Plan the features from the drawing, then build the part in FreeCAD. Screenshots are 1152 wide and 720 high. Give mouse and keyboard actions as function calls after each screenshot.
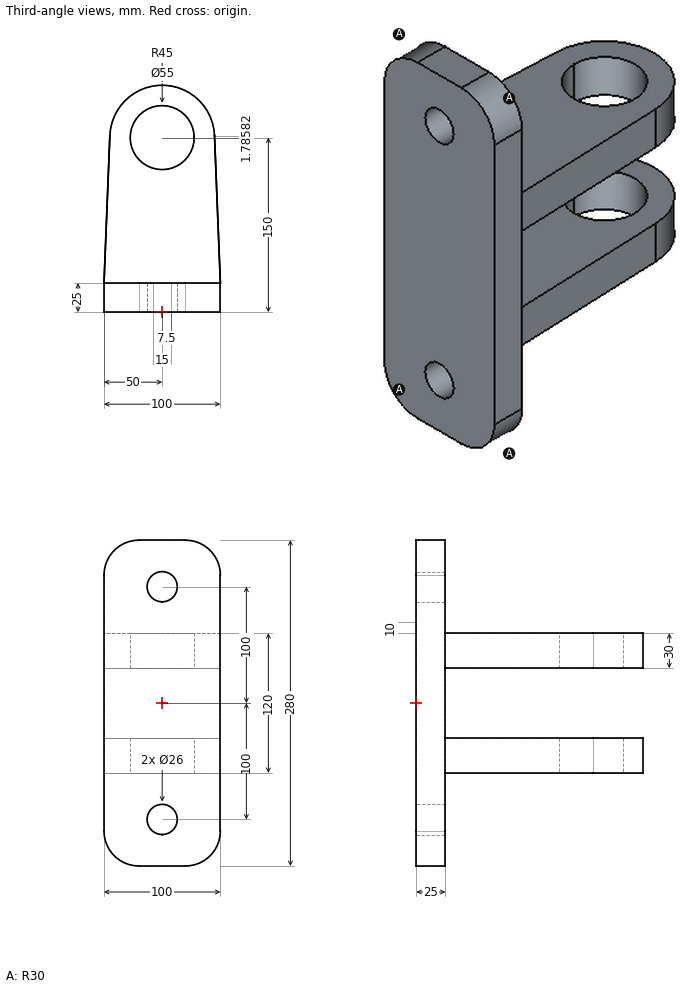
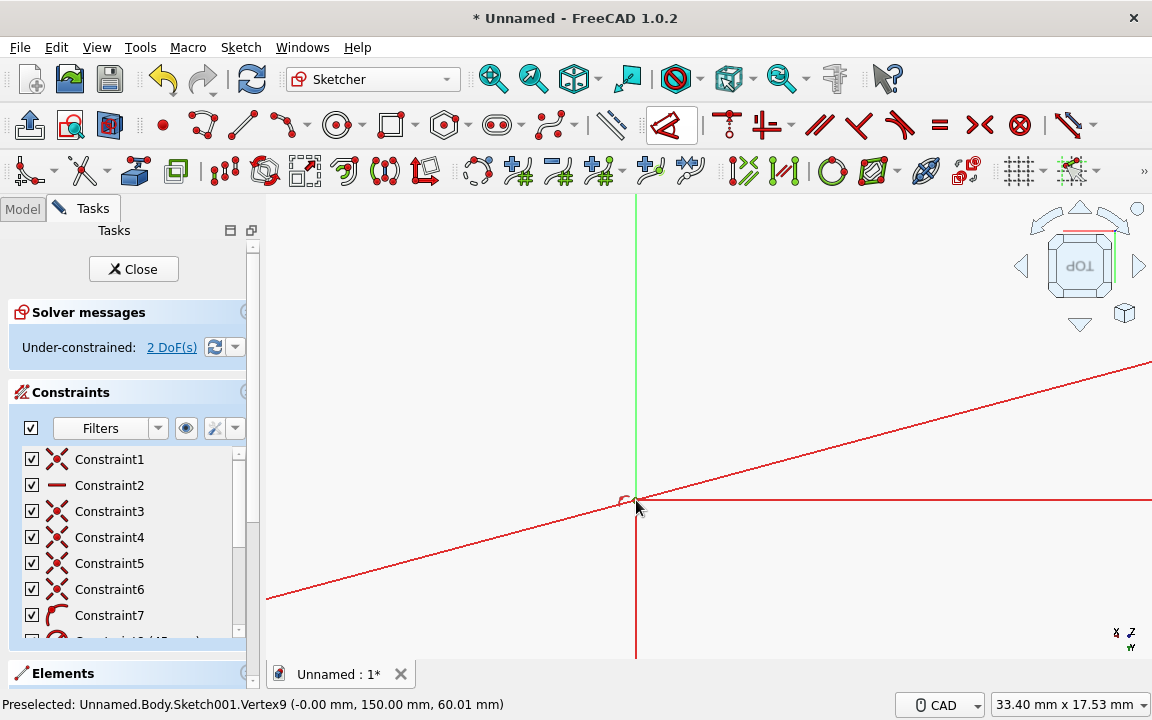
click(692, 126)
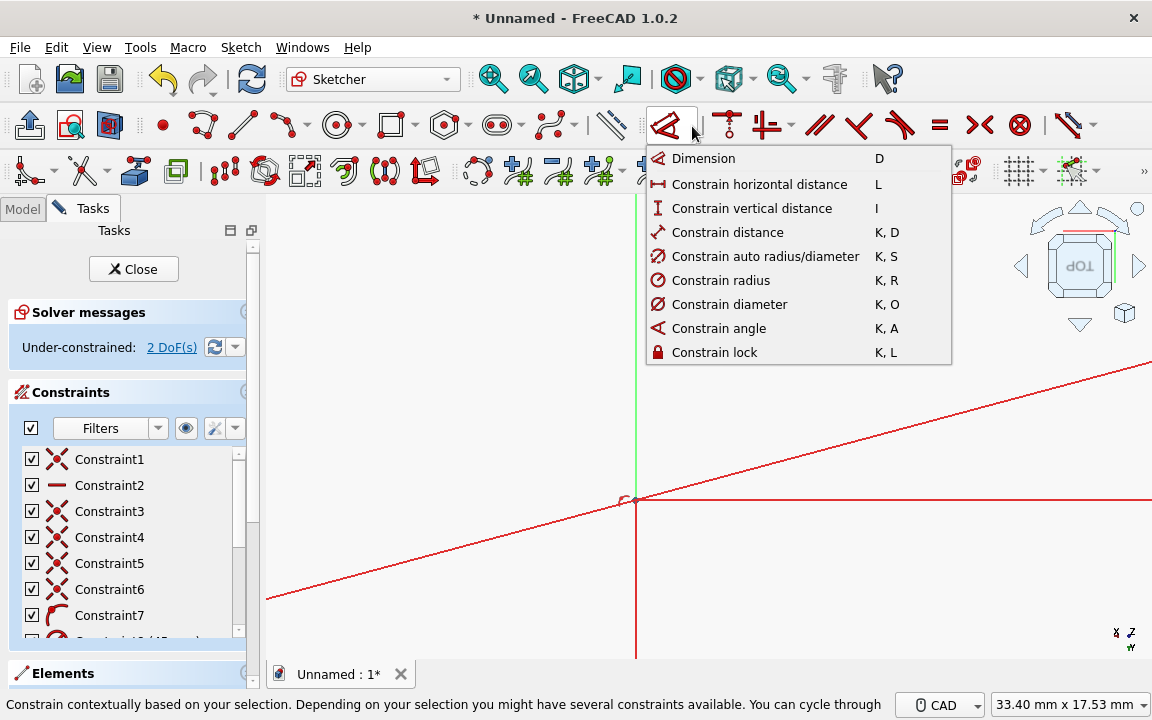
click(799, 208)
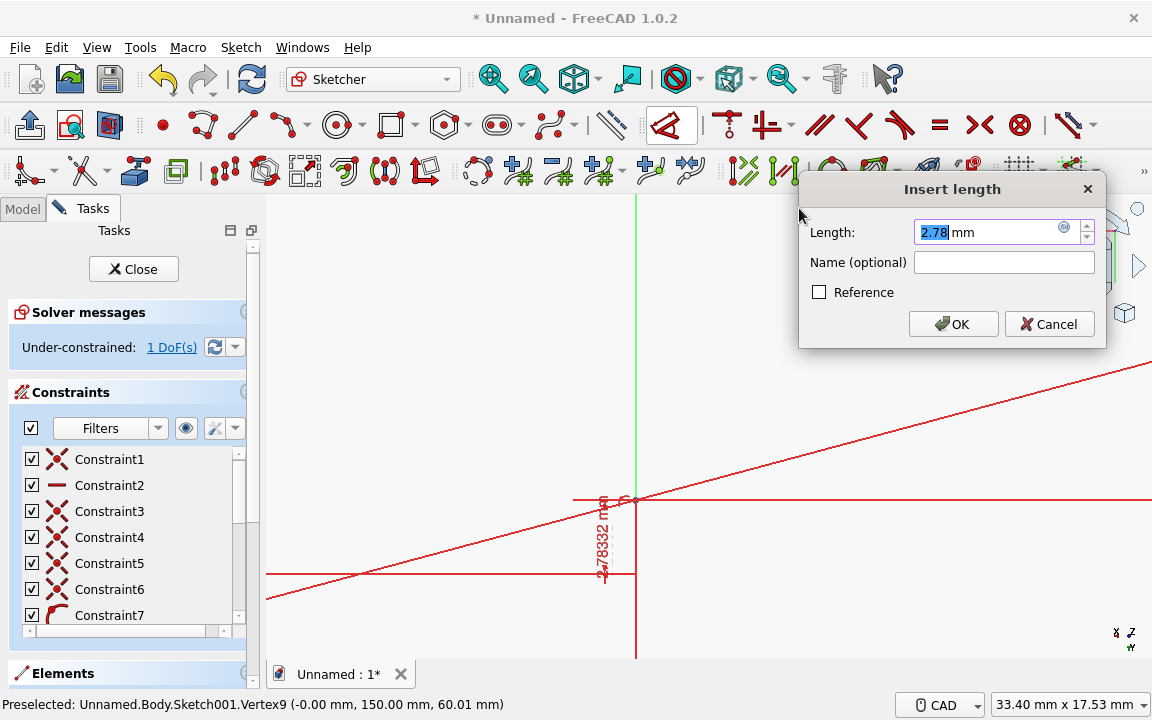
text(1.78582)
key(Return)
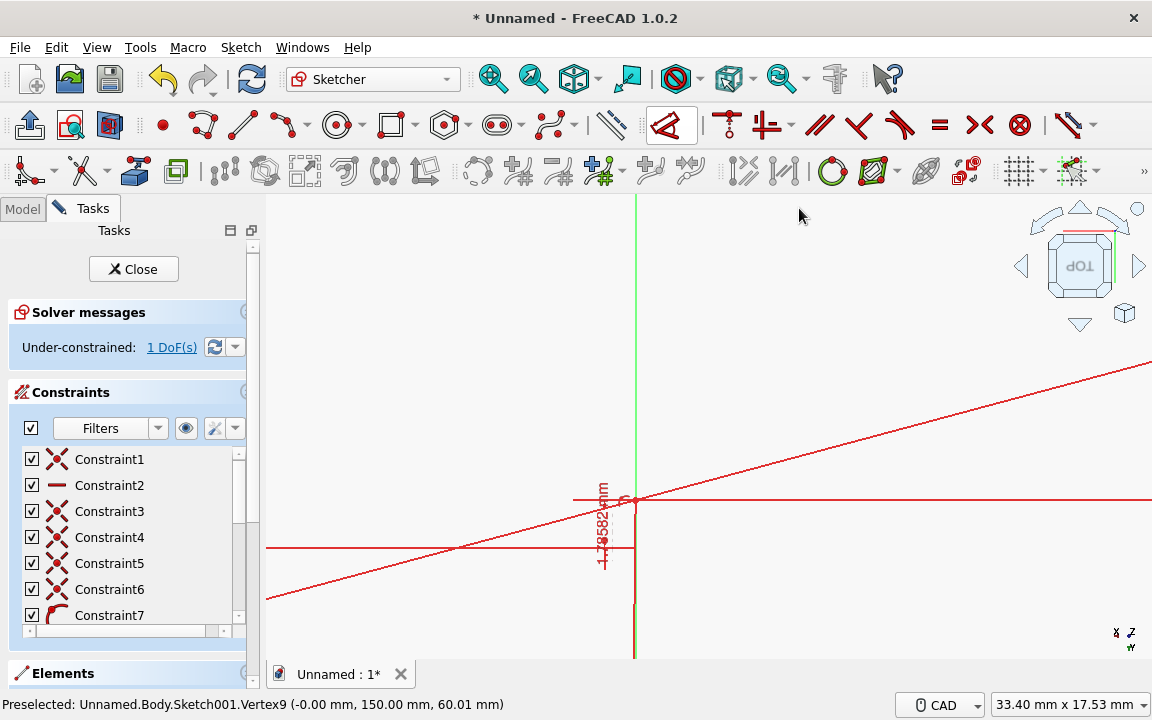
scroll(641, 512, down, 14)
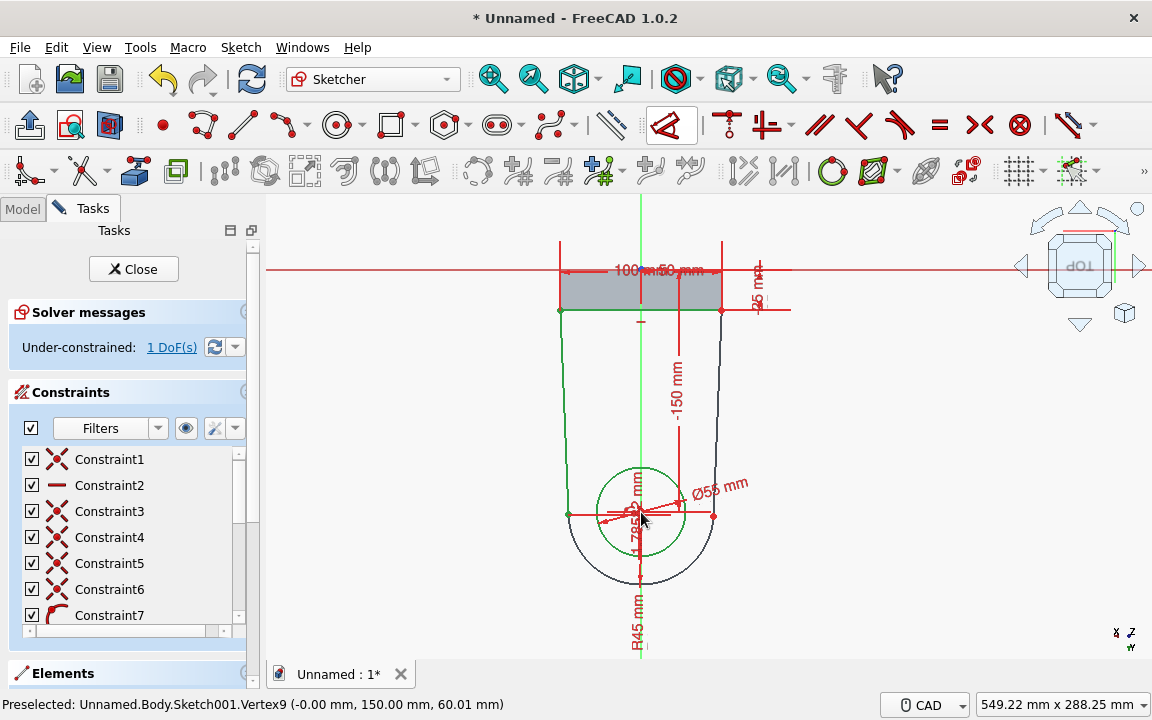
scroll(714, 516, up, 14)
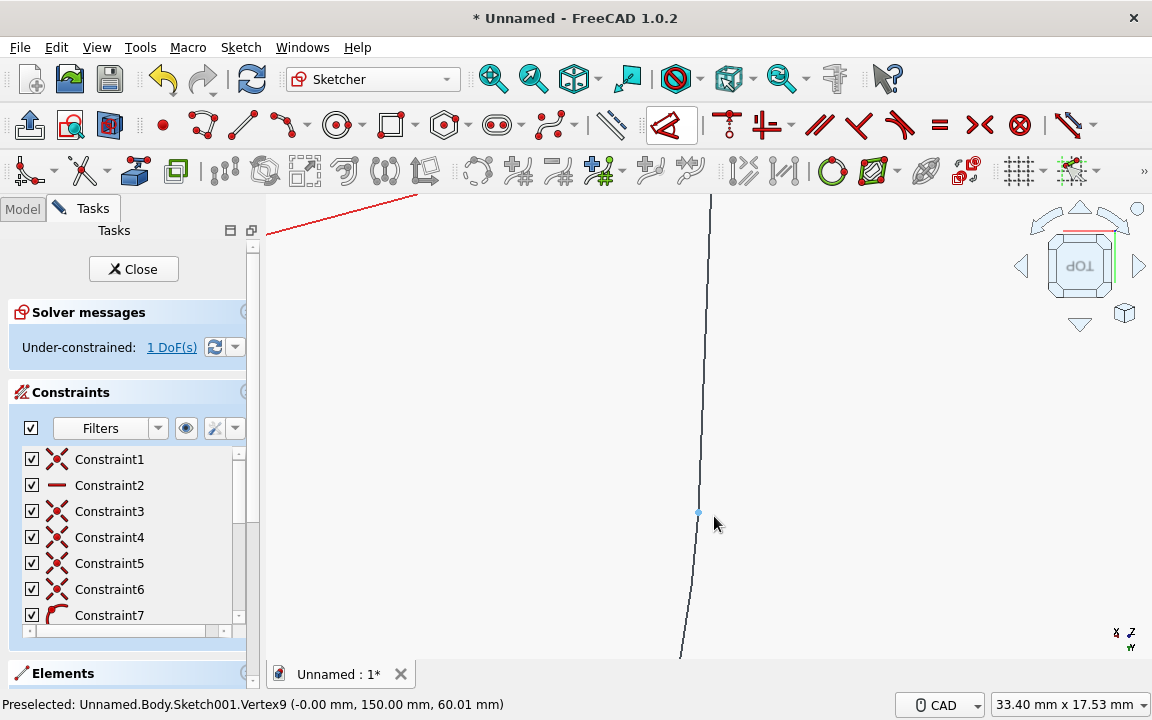
click(698, 512)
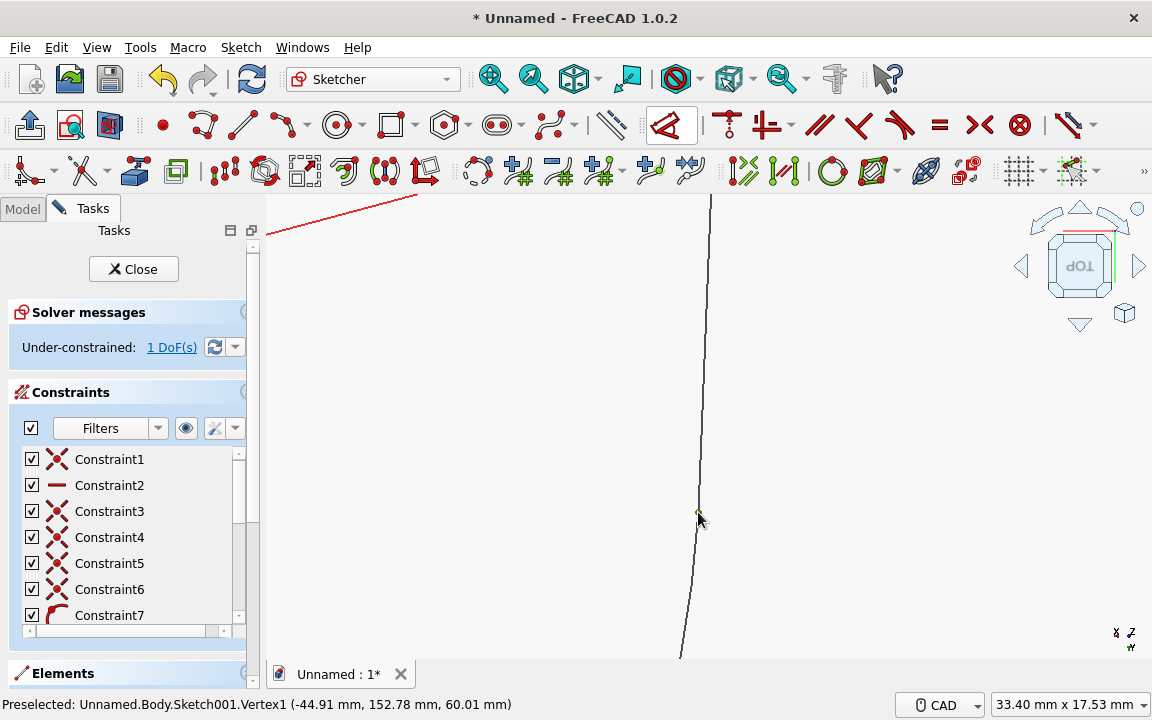
scroll(714, 516, down, 14)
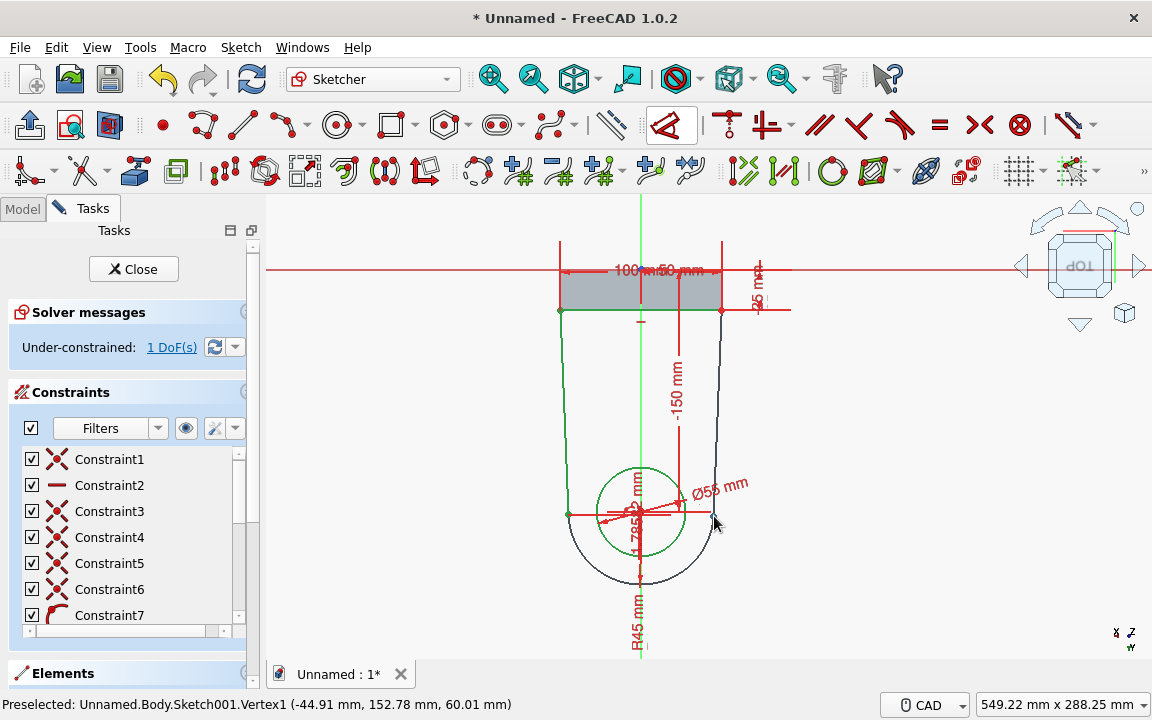
scroll(641, 512, up, 14)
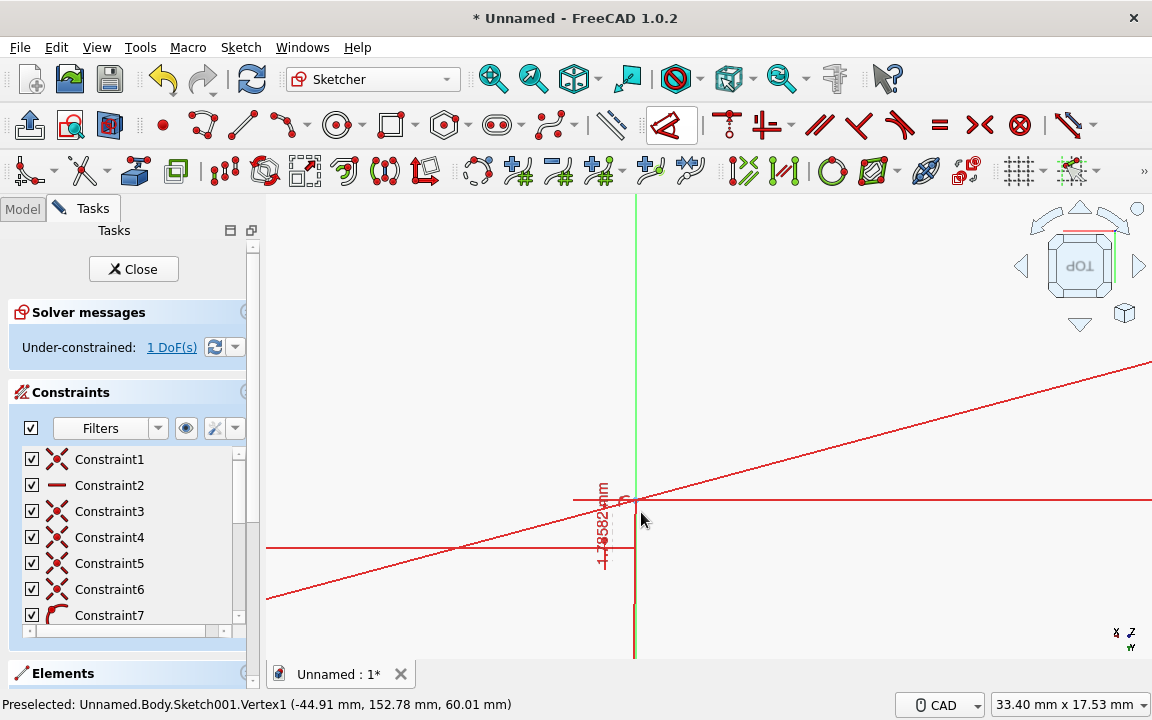
click(636, 500)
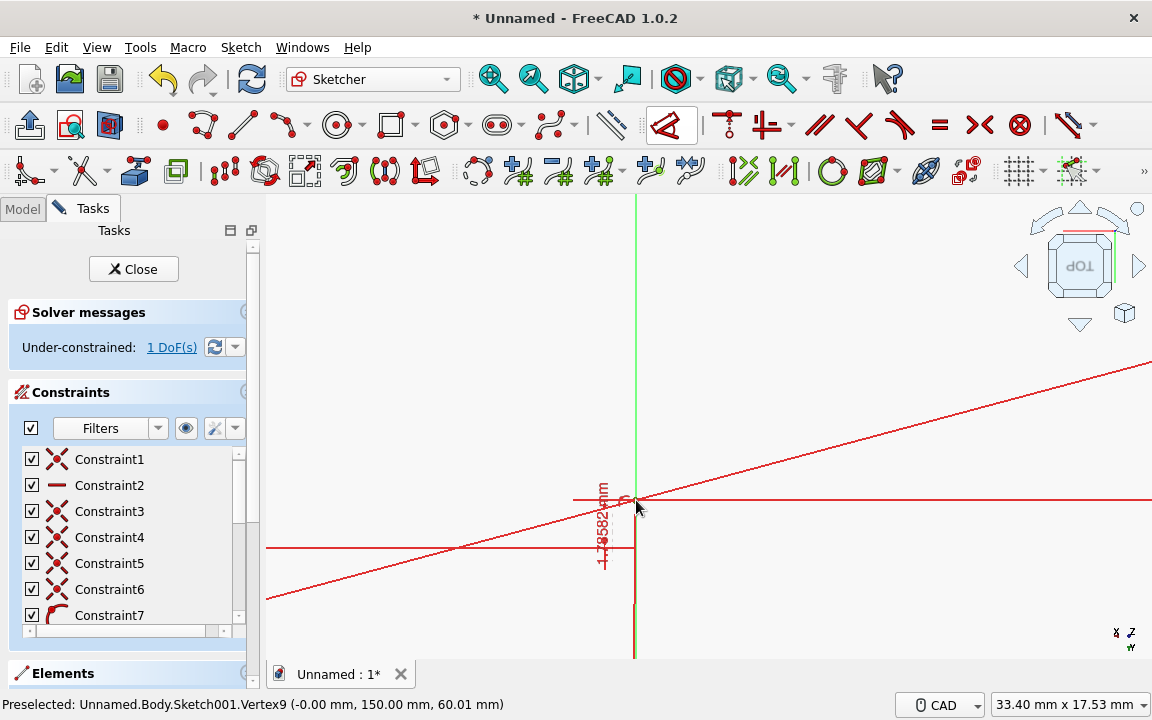
click(692, 126)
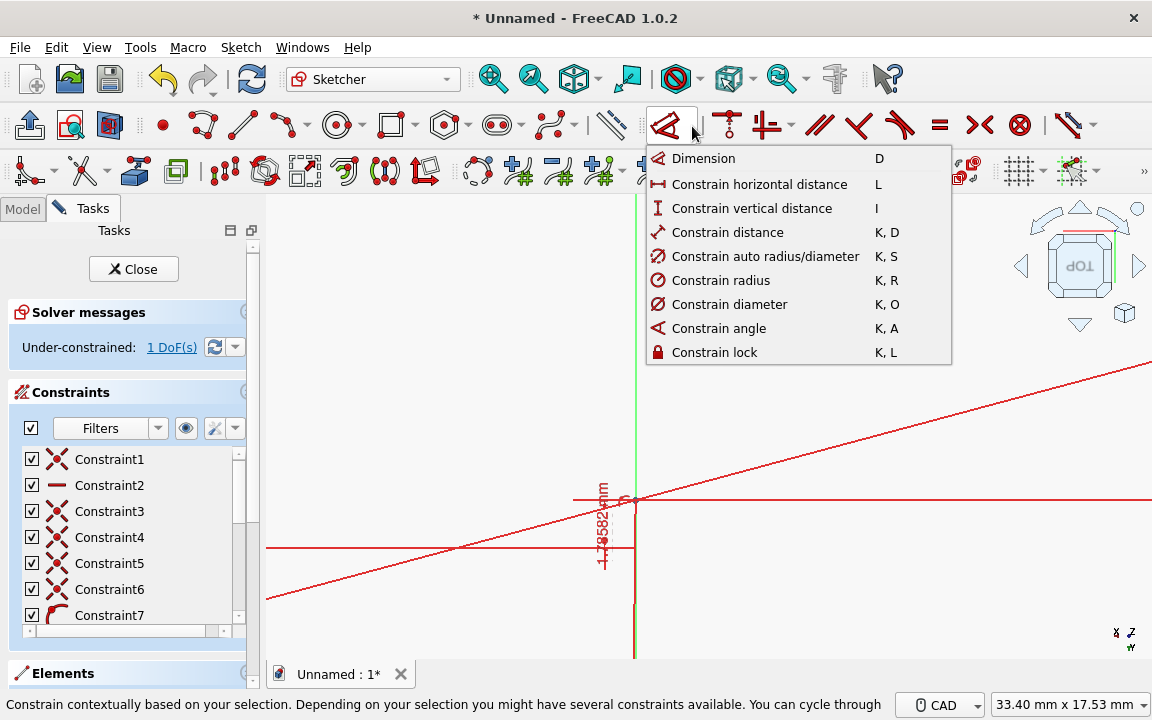
click(799, 208)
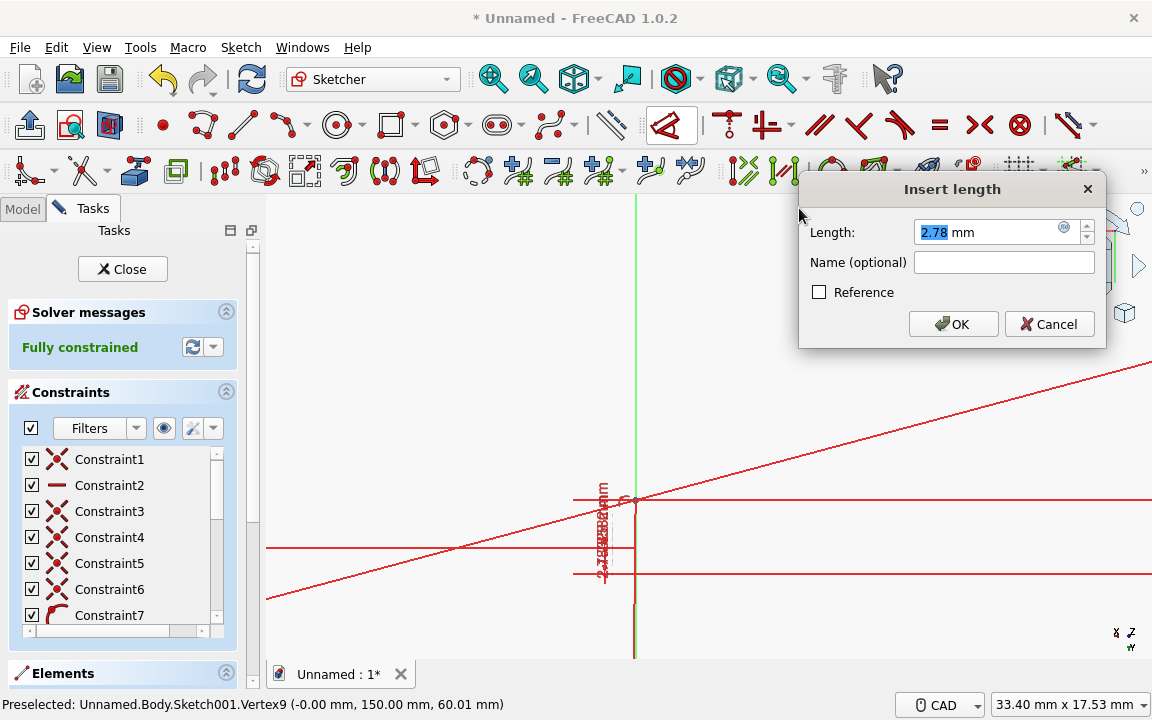
text(1.78582)
key(Return)